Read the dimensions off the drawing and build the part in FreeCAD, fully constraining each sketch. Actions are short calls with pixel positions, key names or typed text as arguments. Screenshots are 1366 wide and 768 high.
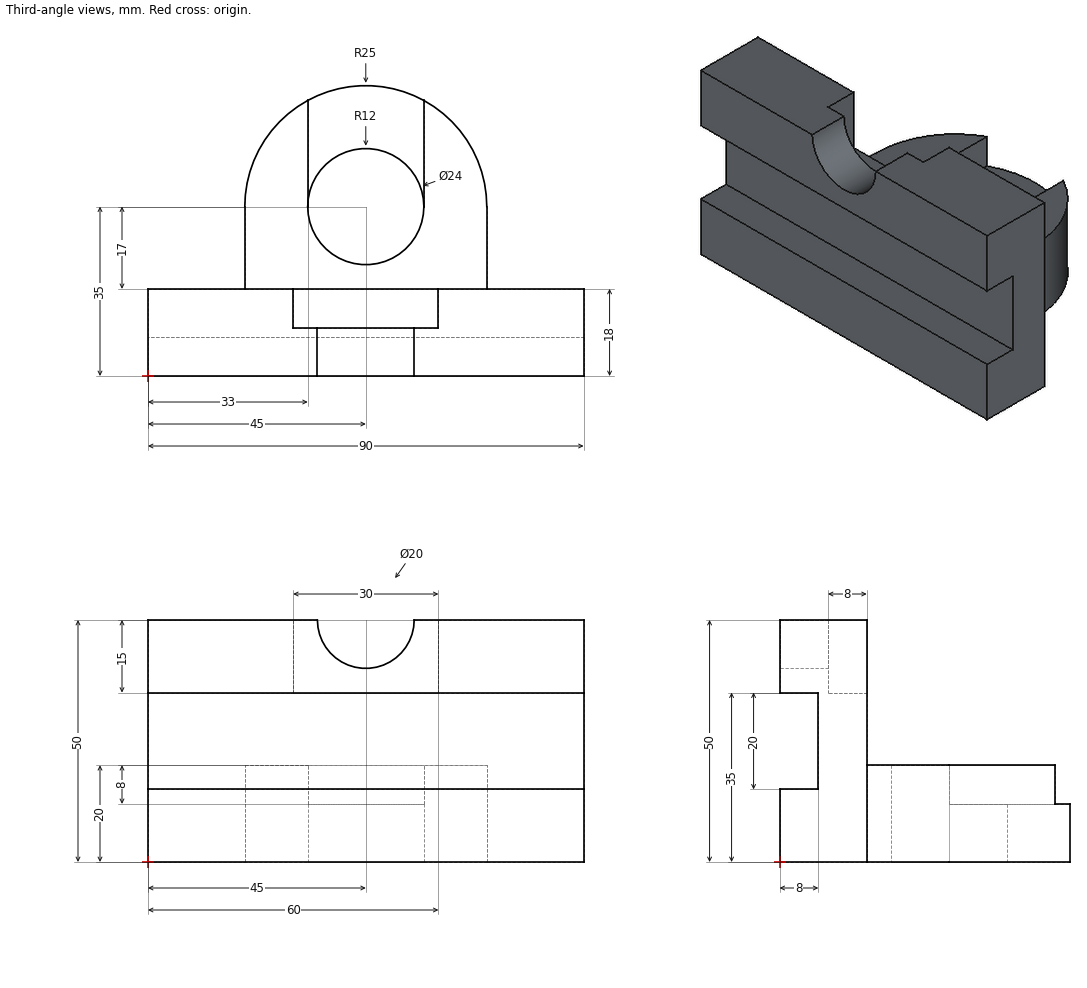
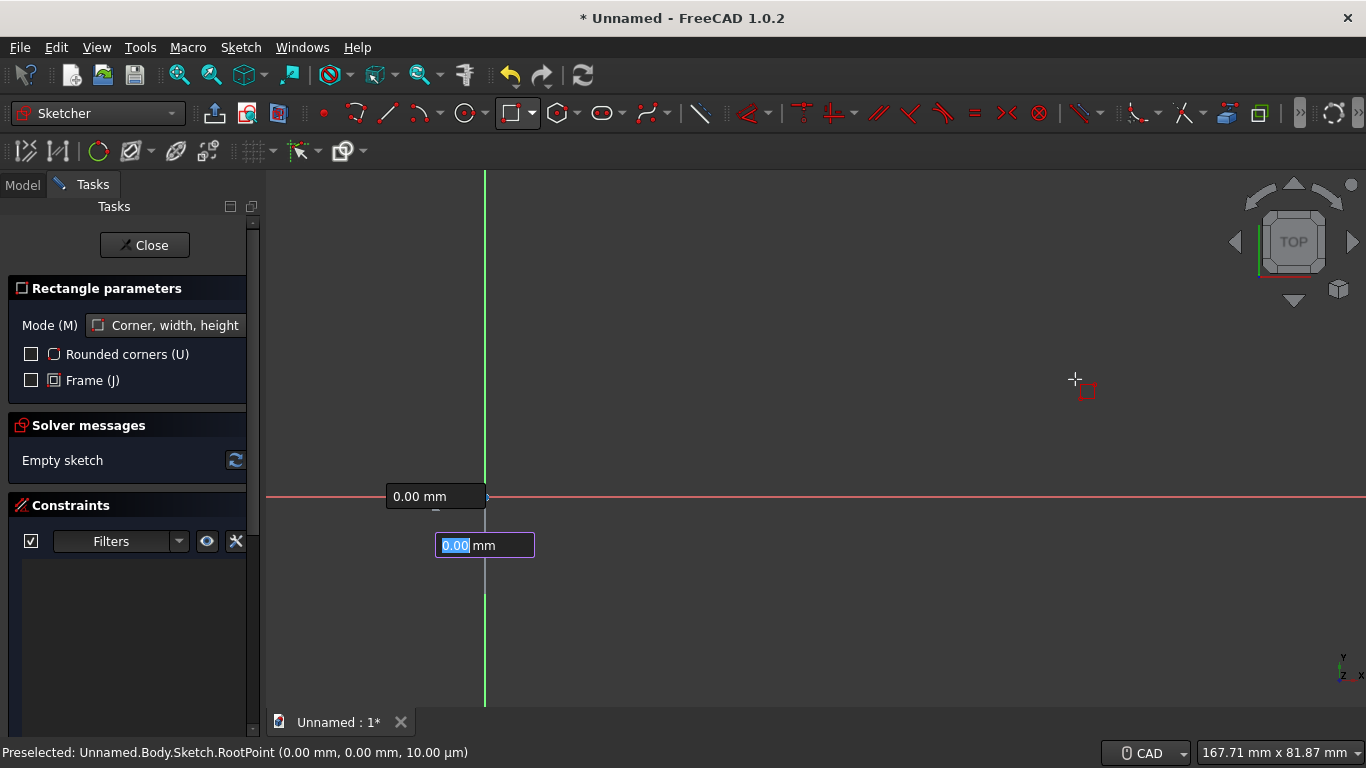
text(90)
key(Tab)
text(18)
key(Return)
key(Escape)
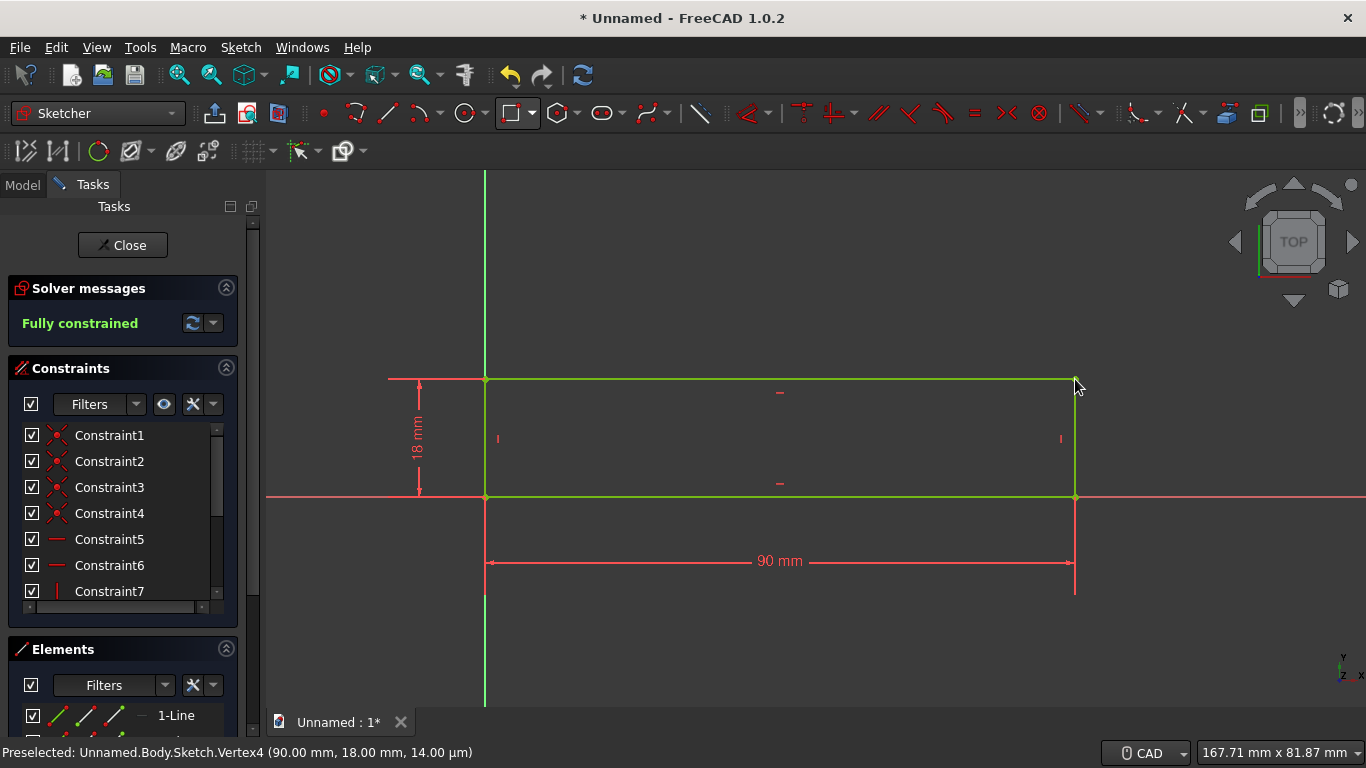
click(123, 245)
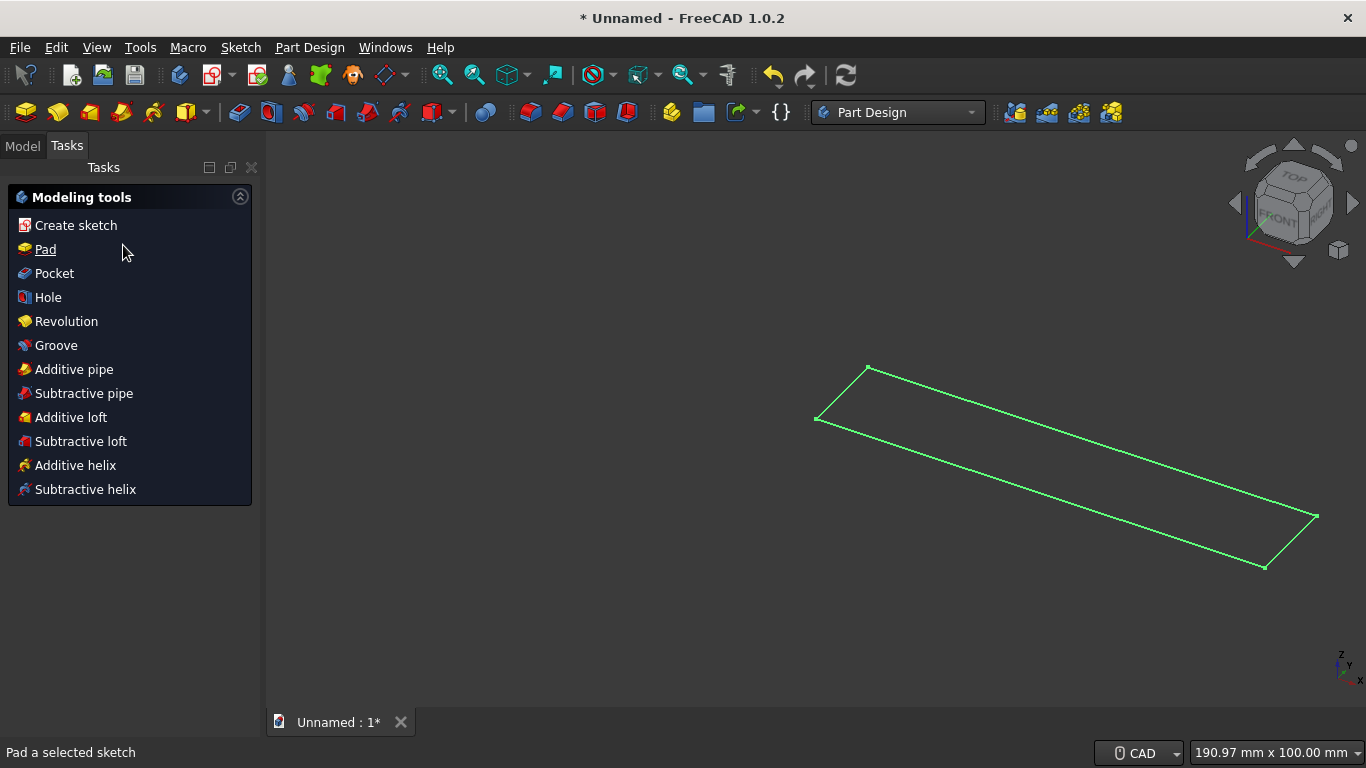
click(26, 112)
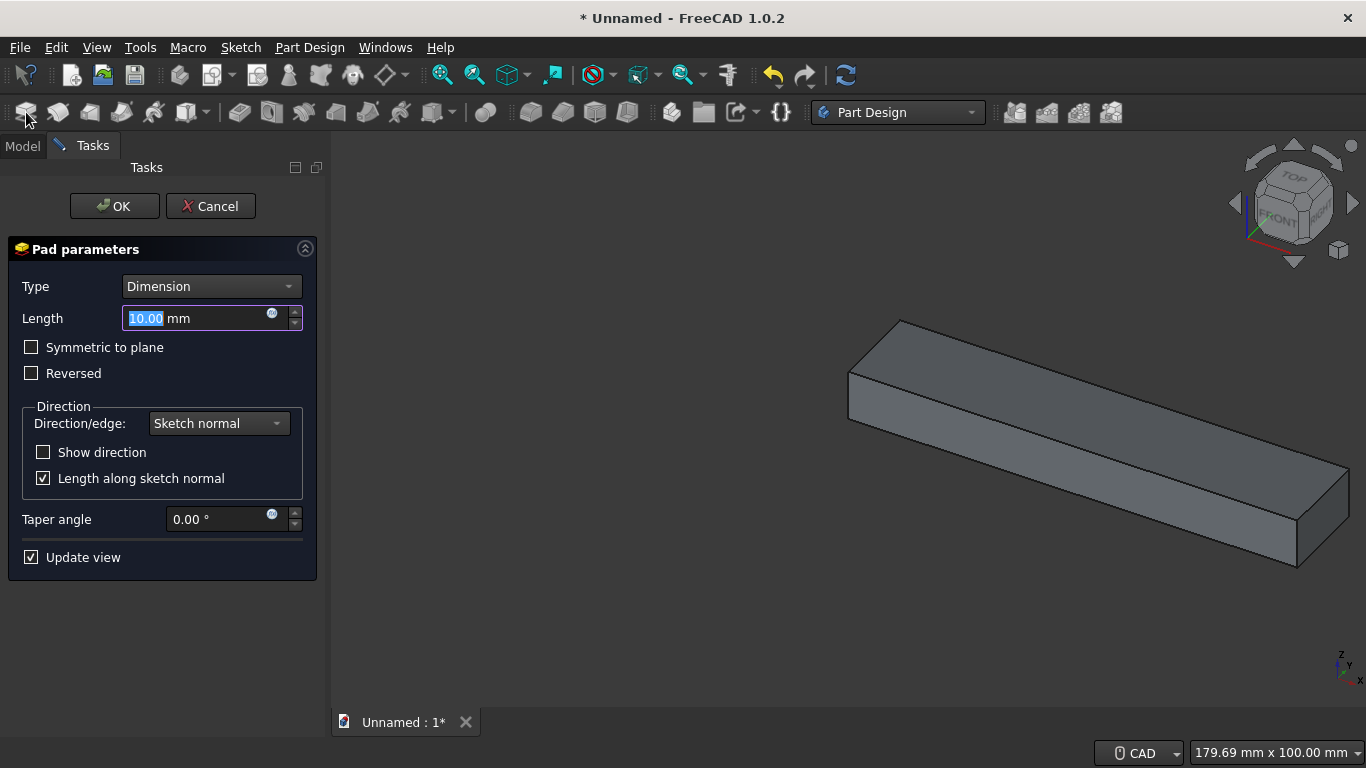
text(50)
key(Tab)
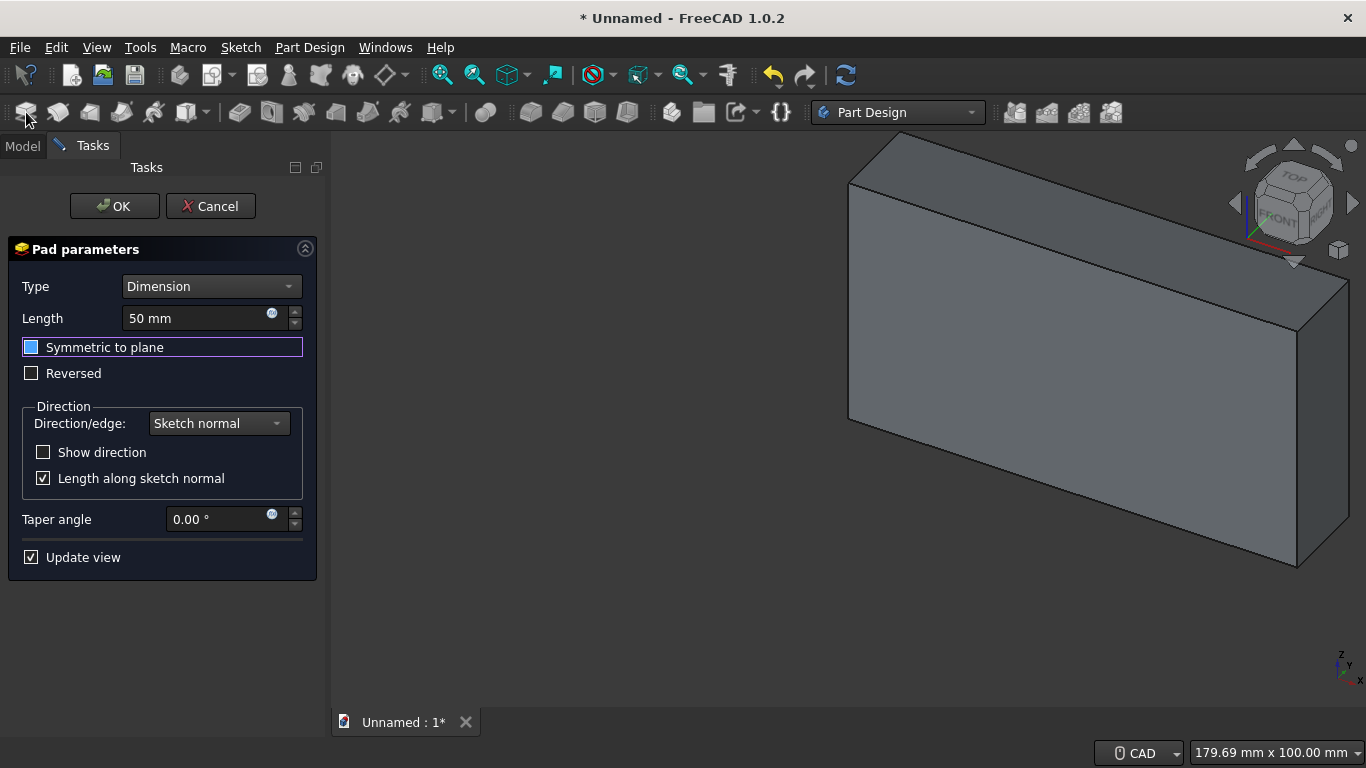
click(115, 206)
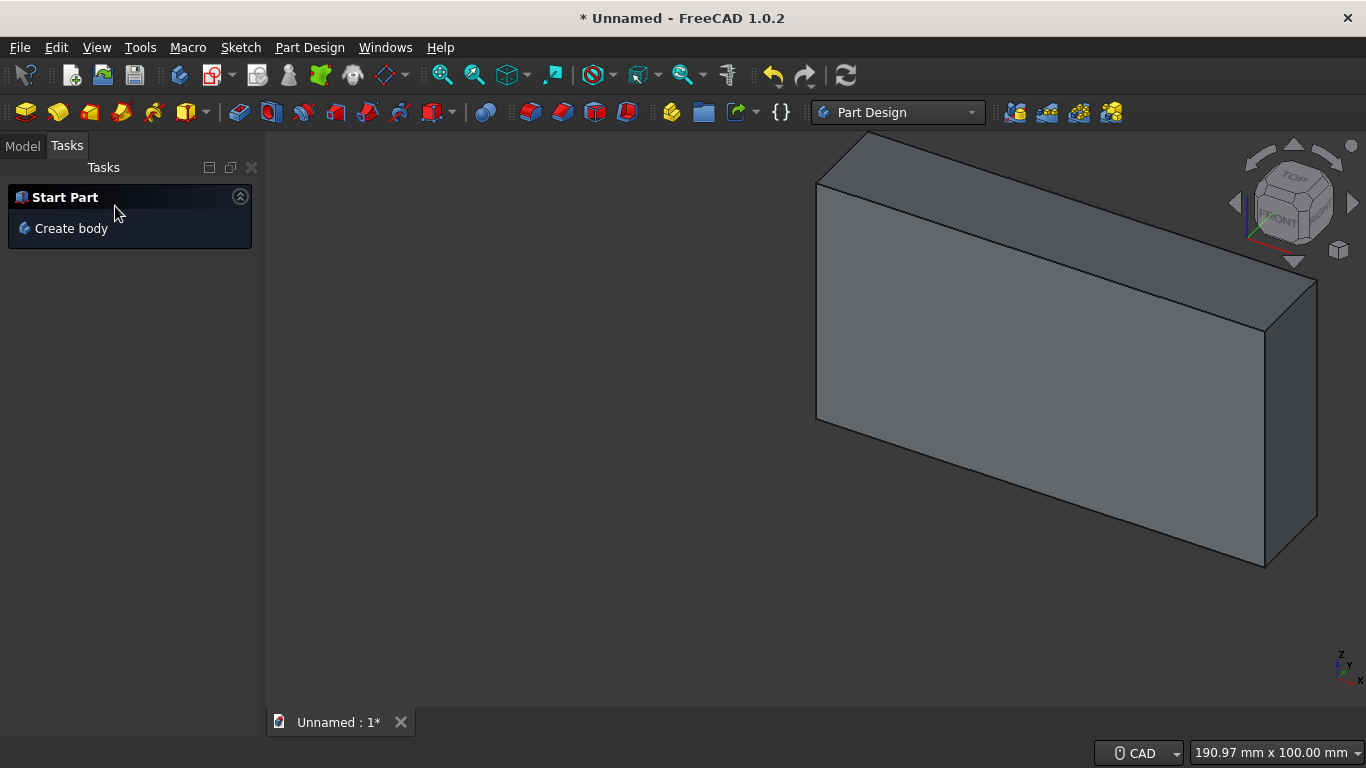
key(5)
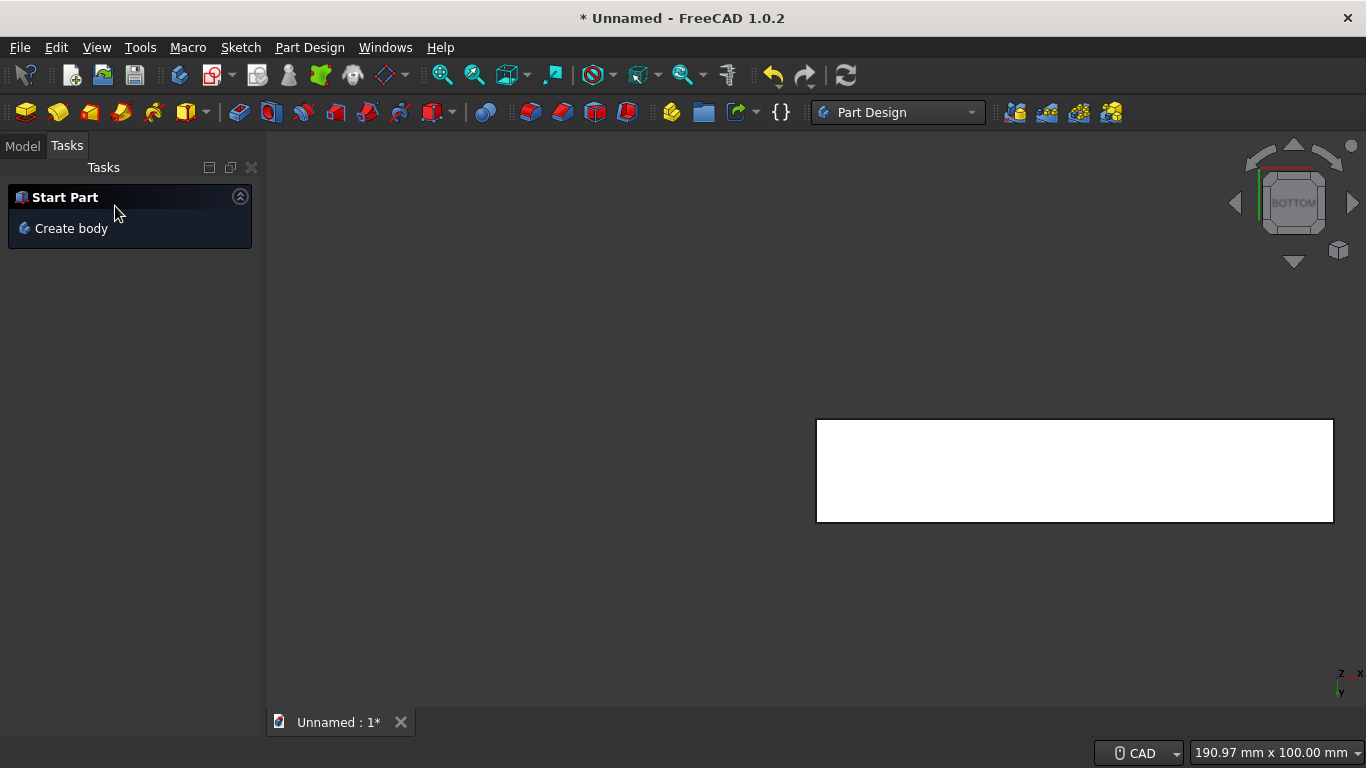
click(1223, 470)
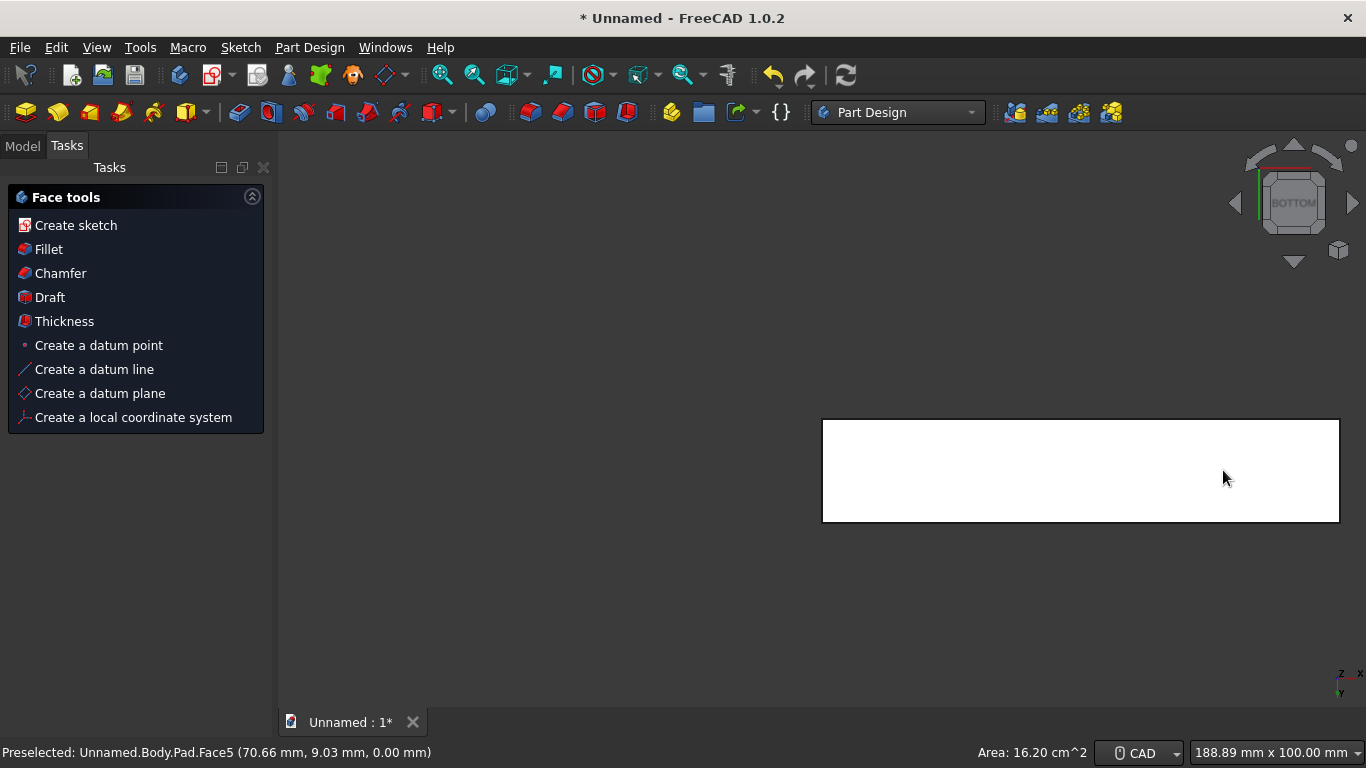
click(212, 76)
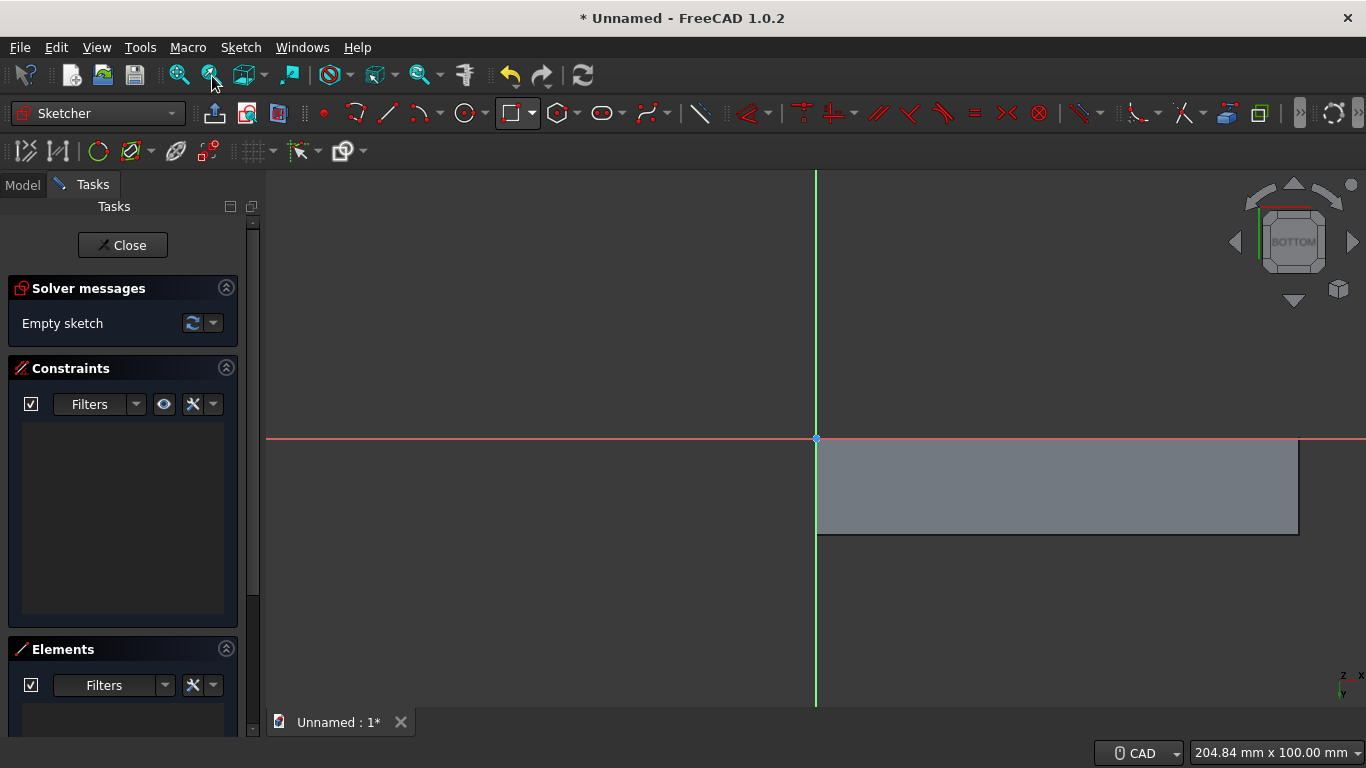
scroll(294, 198, down, 2)